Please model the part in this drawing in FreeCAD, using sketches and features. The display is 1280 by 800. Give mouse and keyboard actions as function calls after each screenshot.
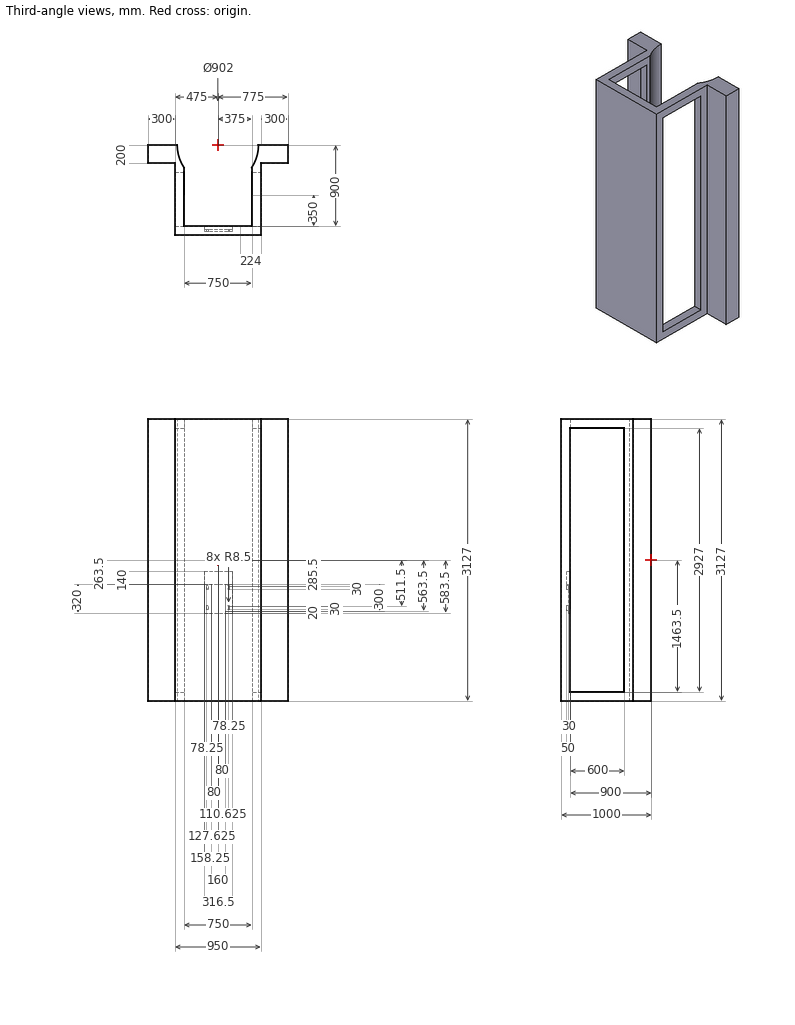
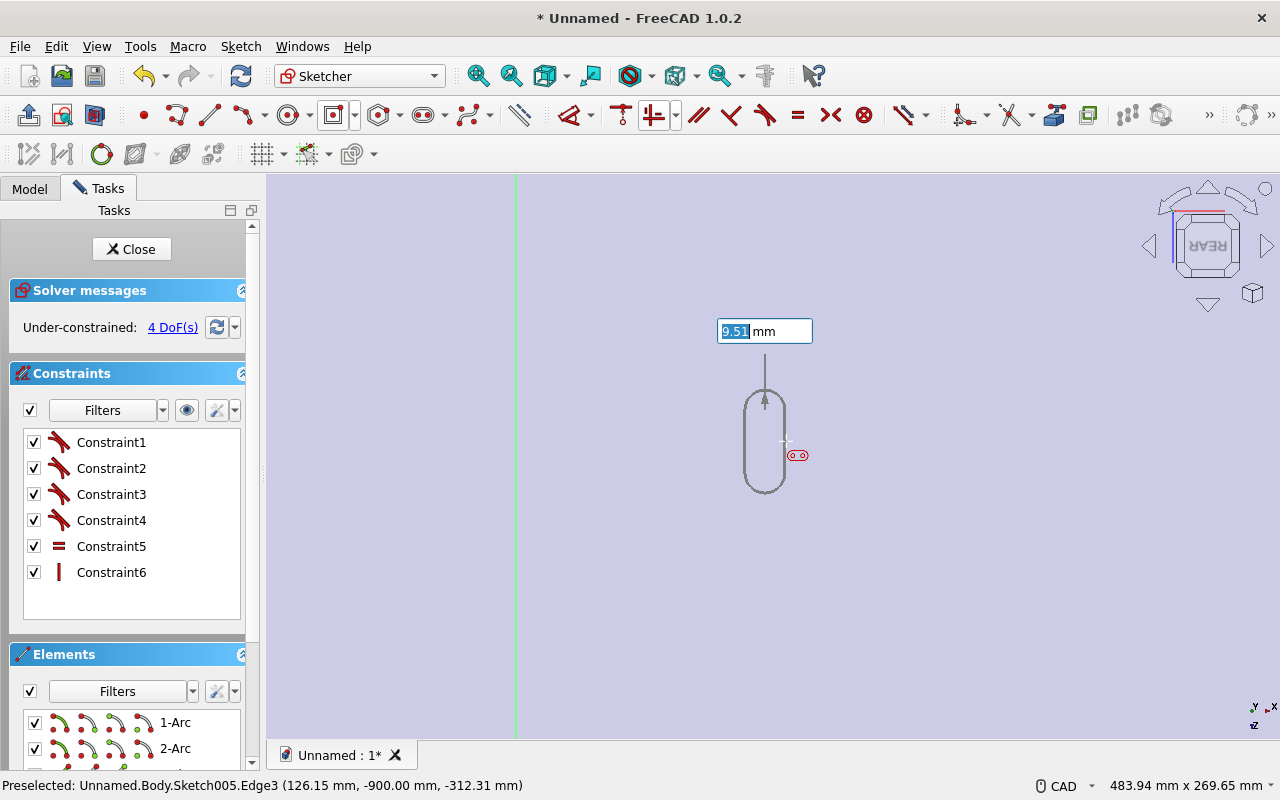
click(783, 439)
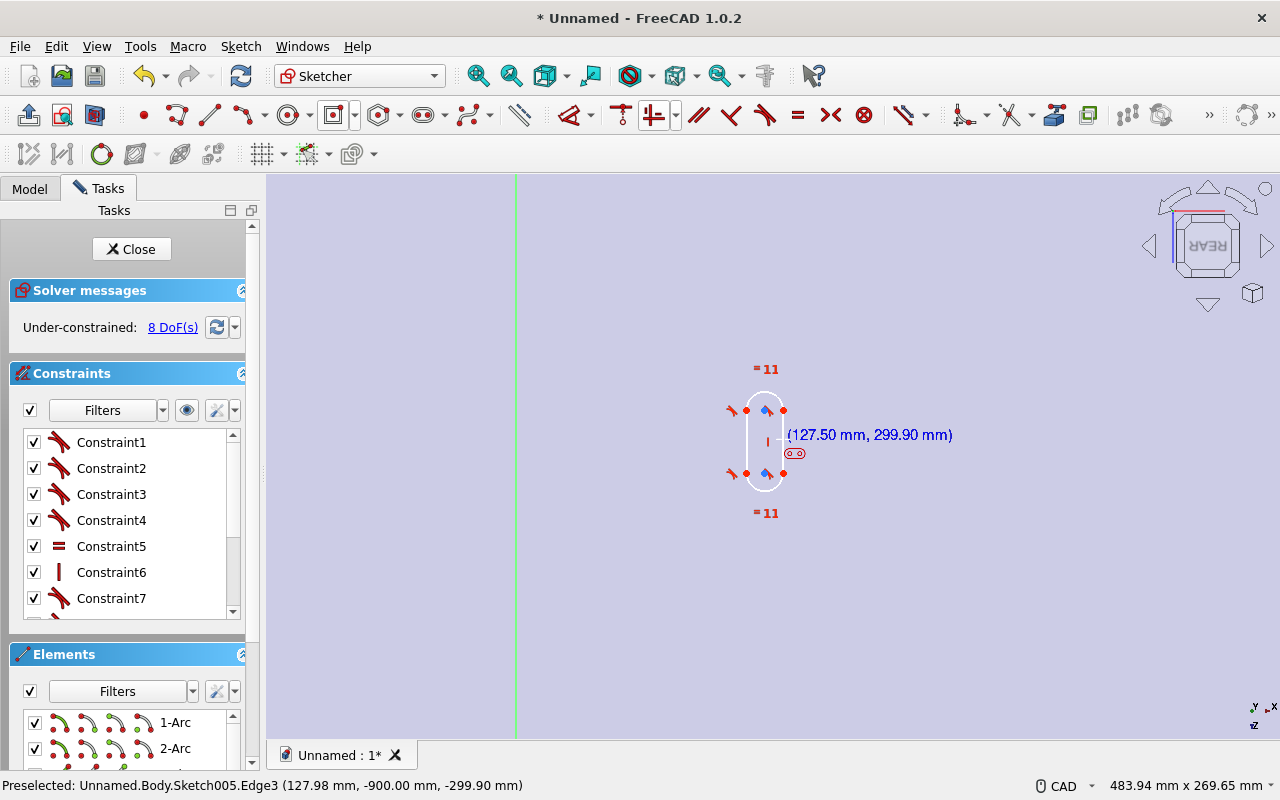
scroll(786, 441, down, 6)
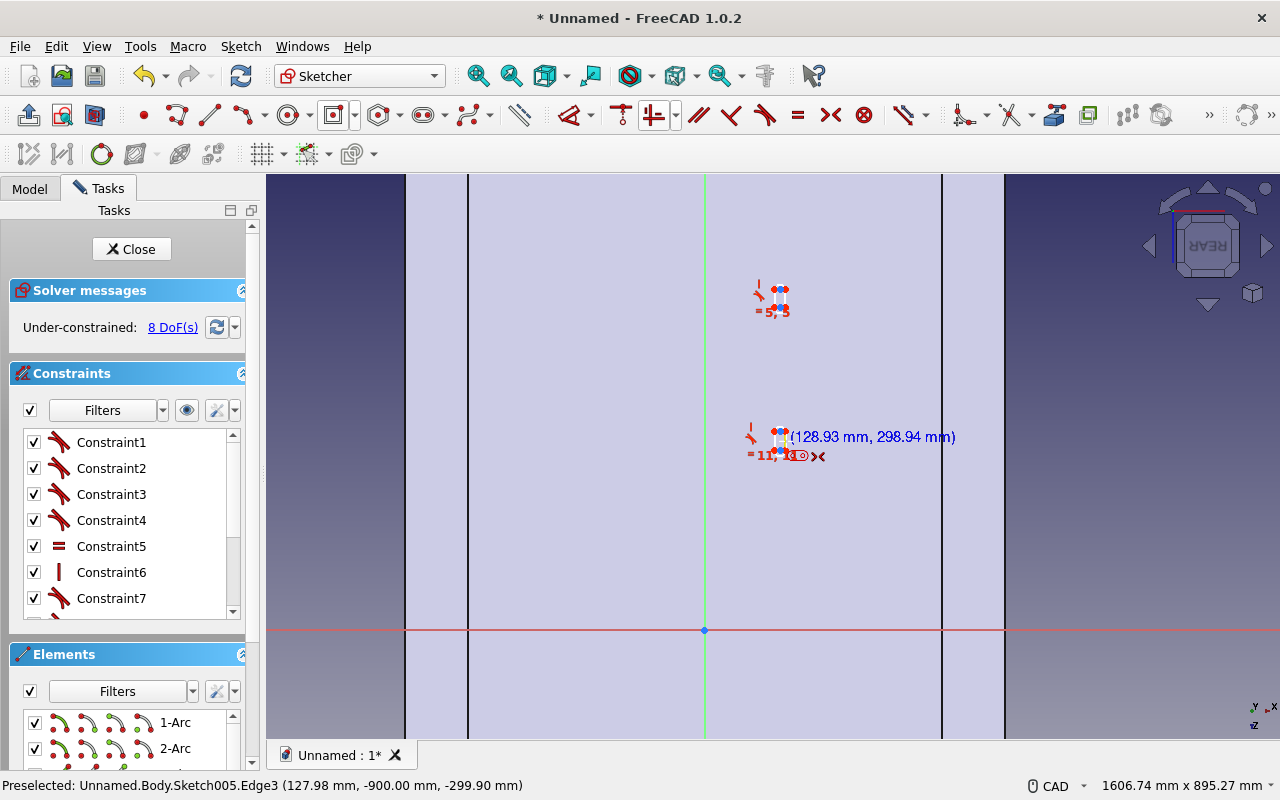
scroll(630, 450, up, 8)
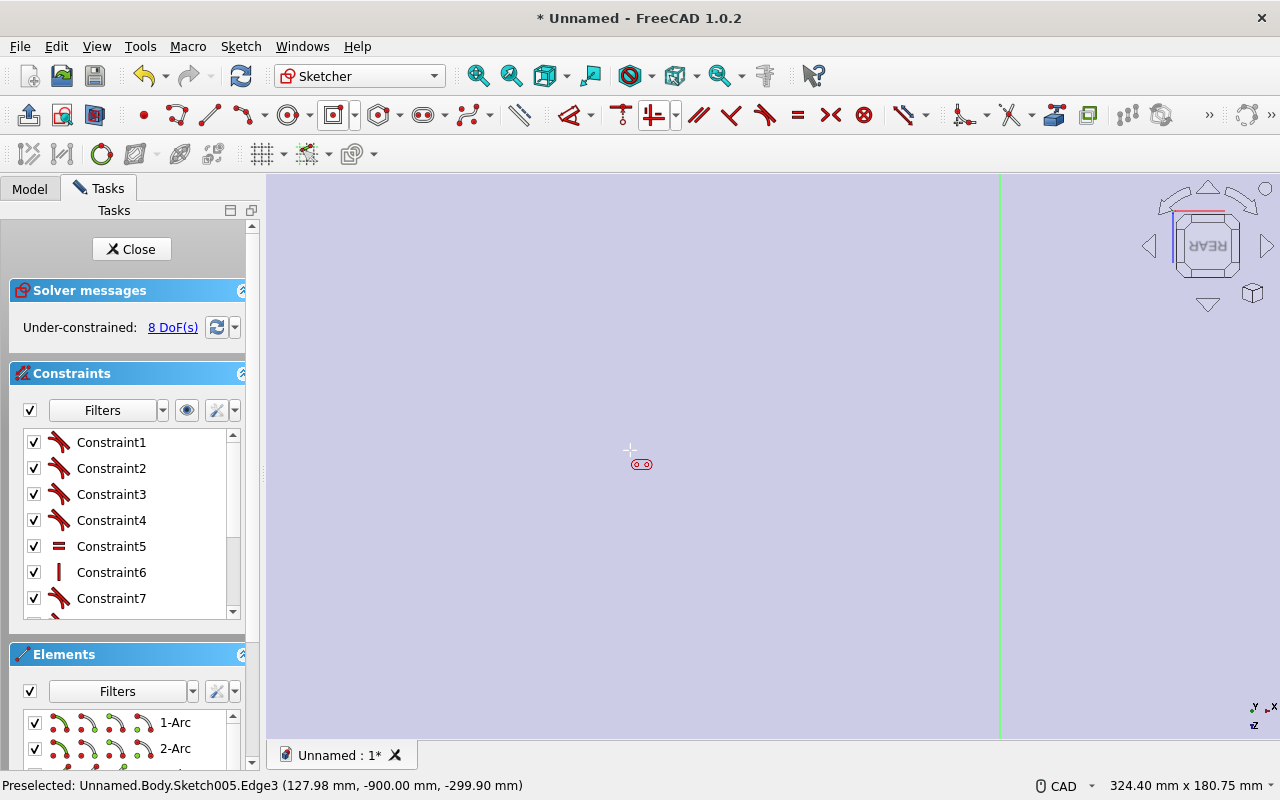
scroll(630, 450, down, 8)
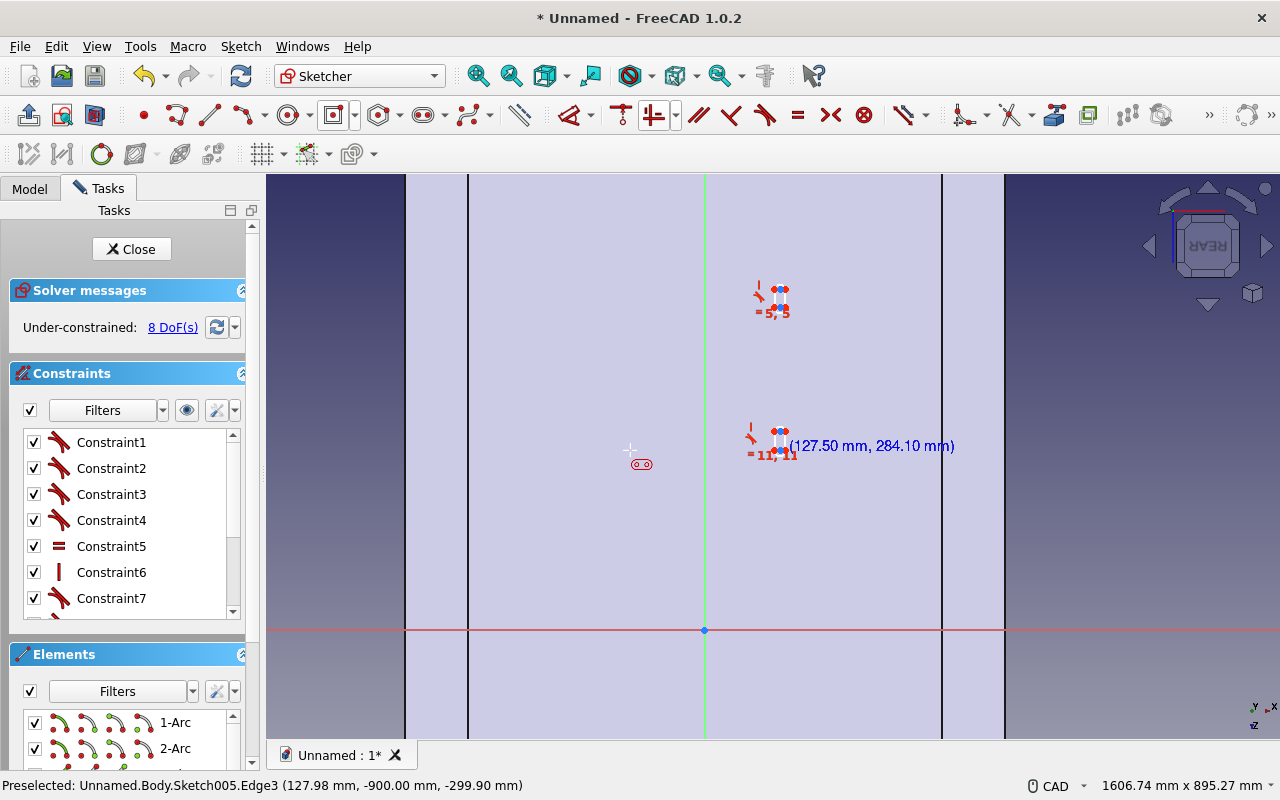
click(630, 450)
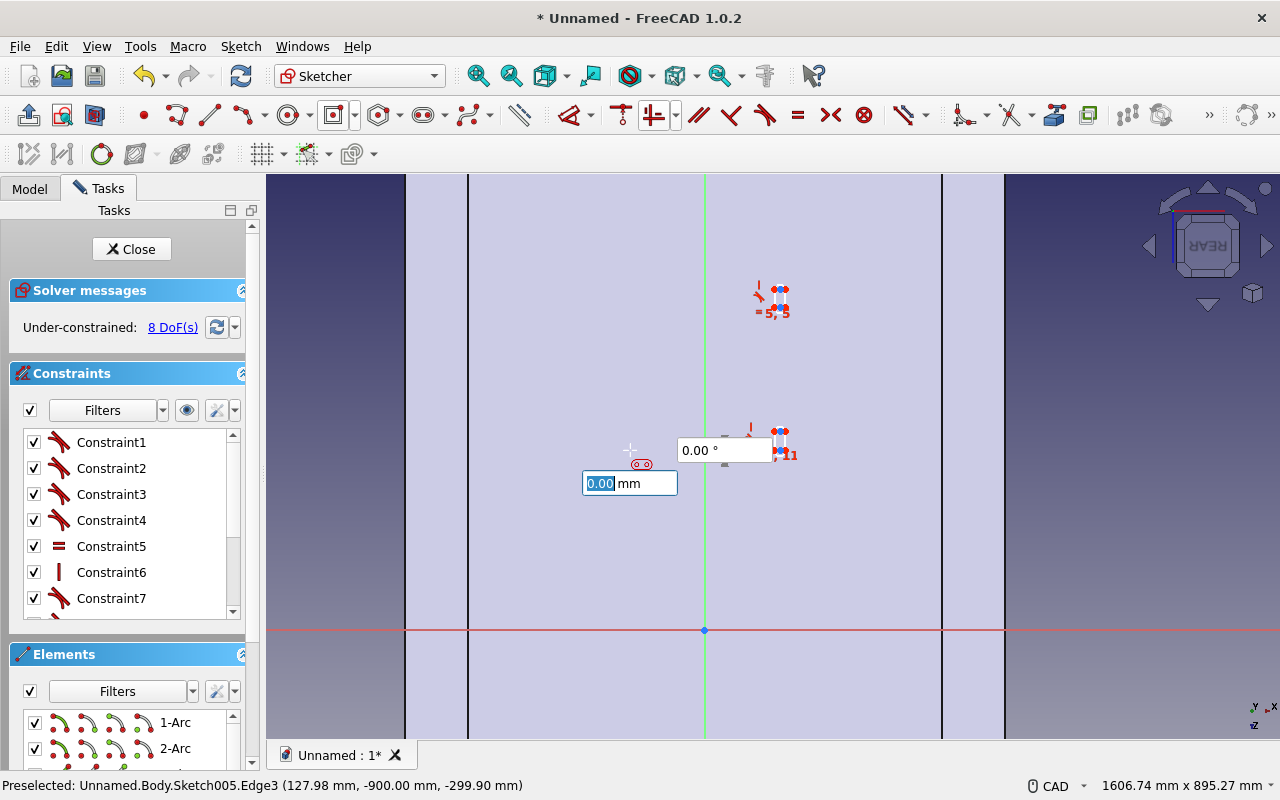
click(630, 431)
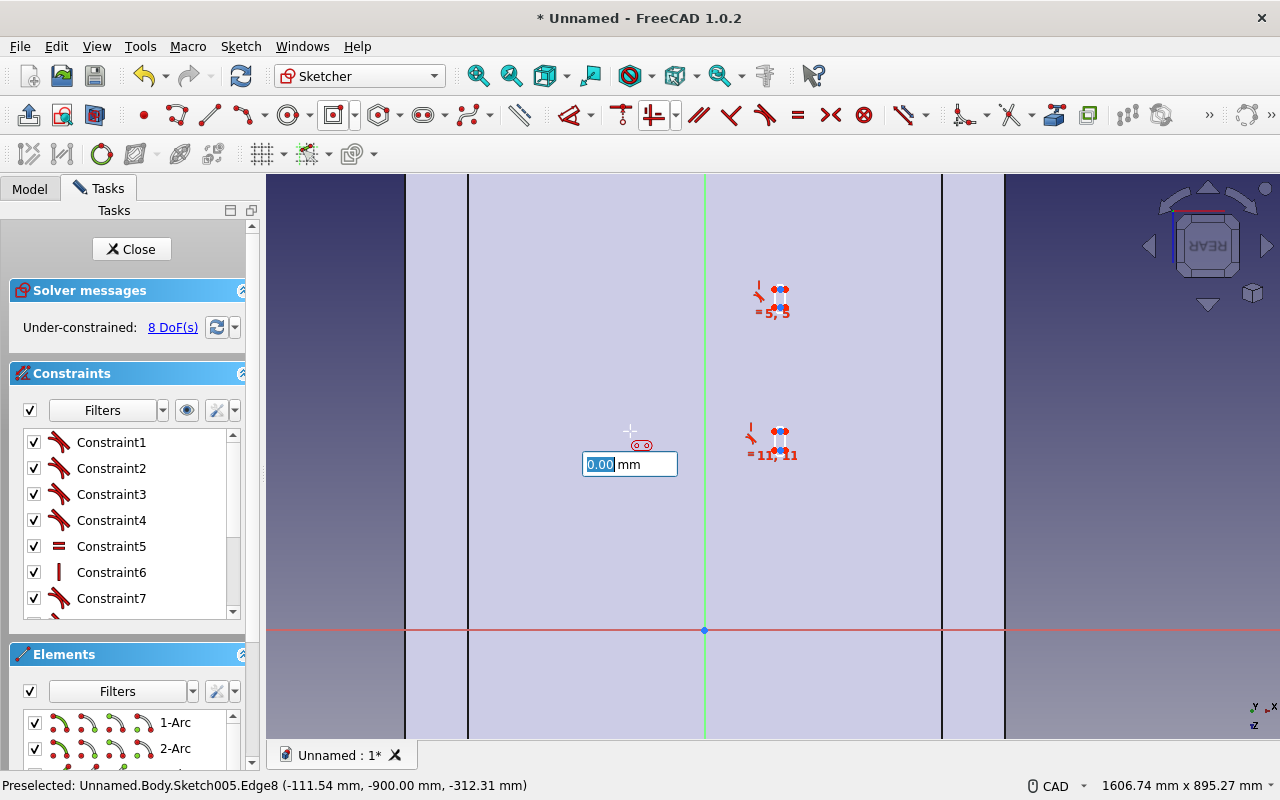
scroll(635, 441, up, 6)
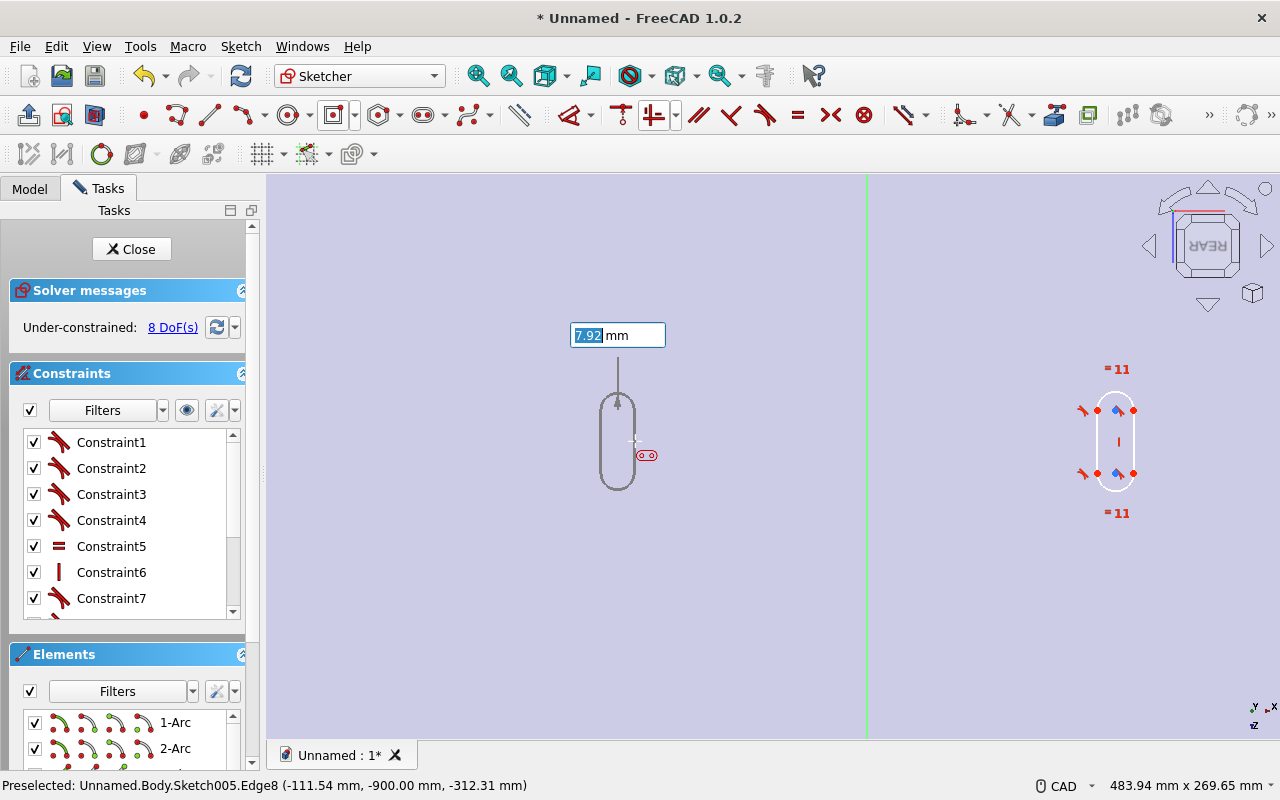
click(635, 439)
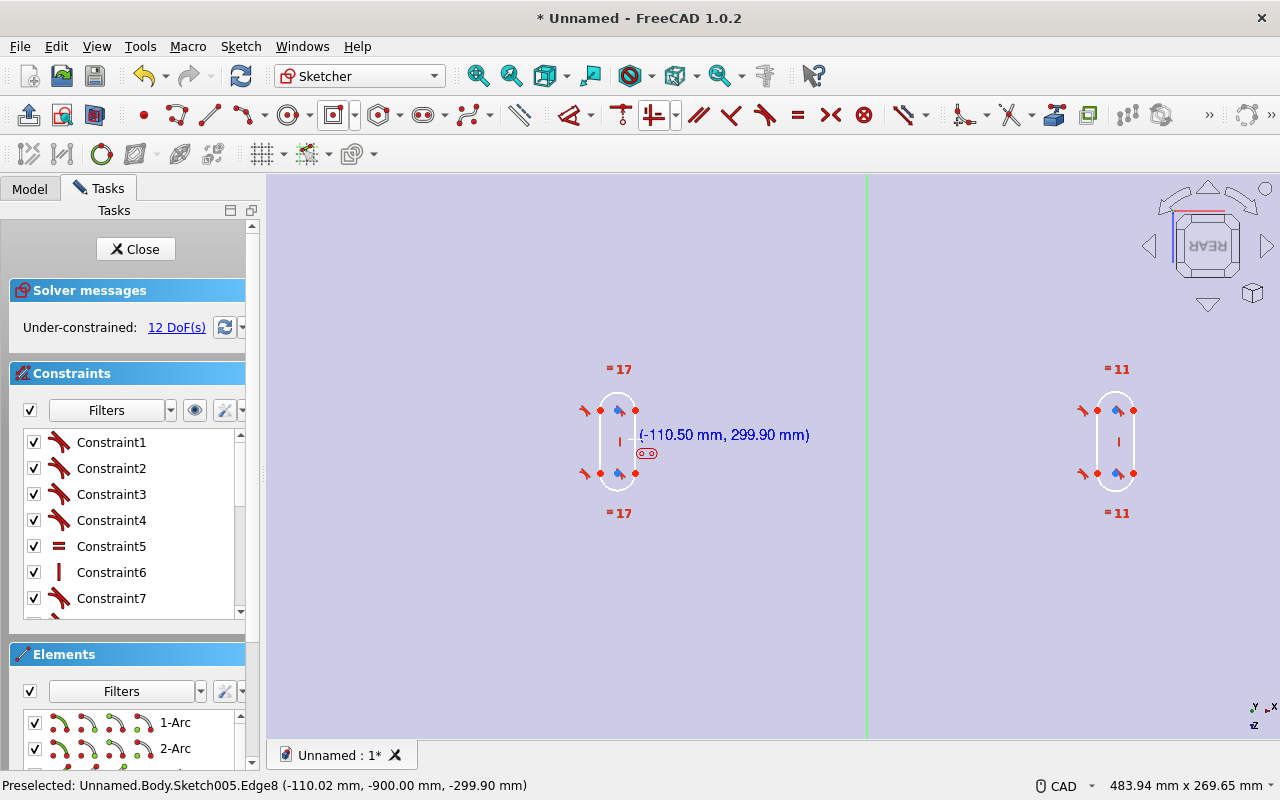
scroll(635, 441, down, 6)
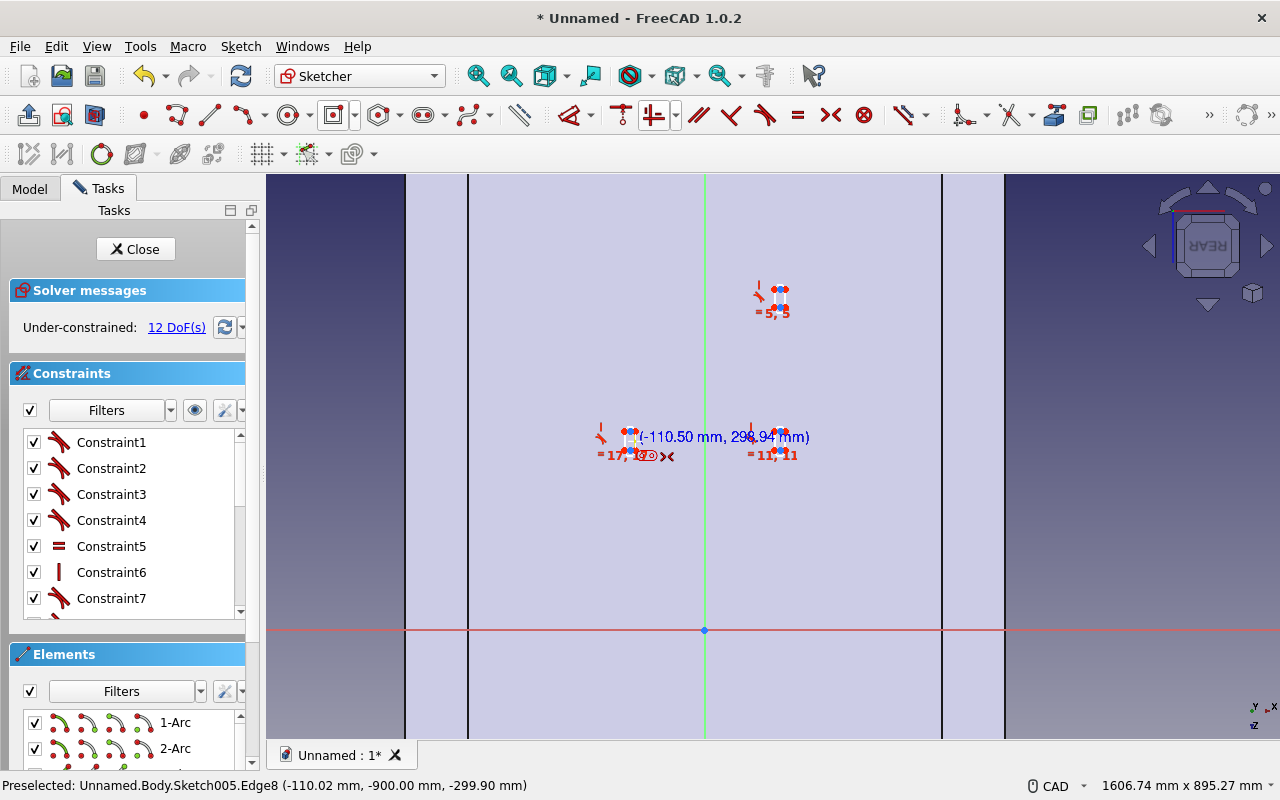
scroll(630, 307, up, 8)